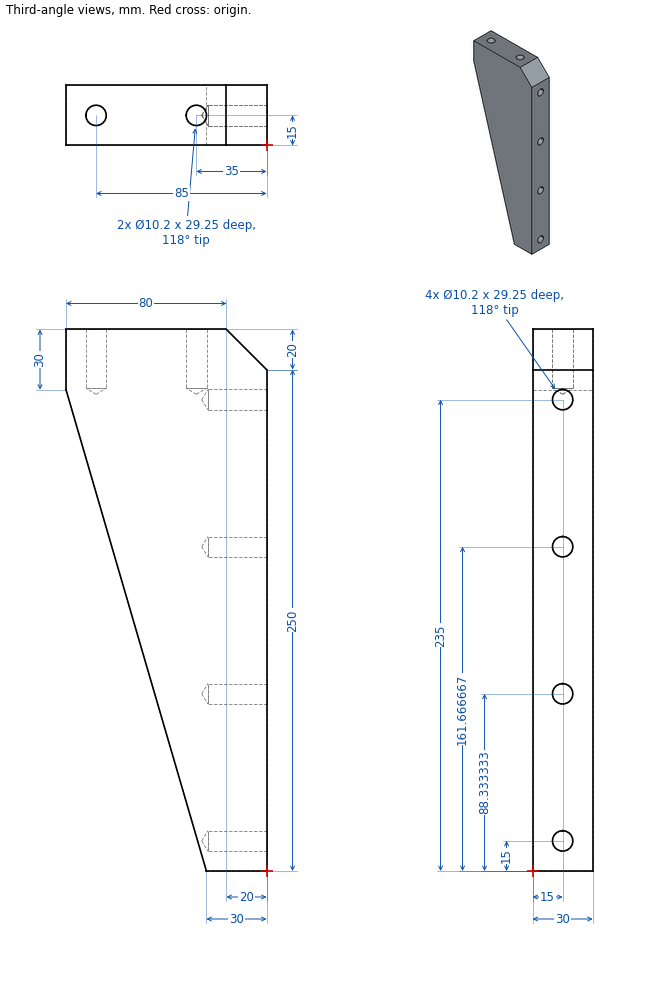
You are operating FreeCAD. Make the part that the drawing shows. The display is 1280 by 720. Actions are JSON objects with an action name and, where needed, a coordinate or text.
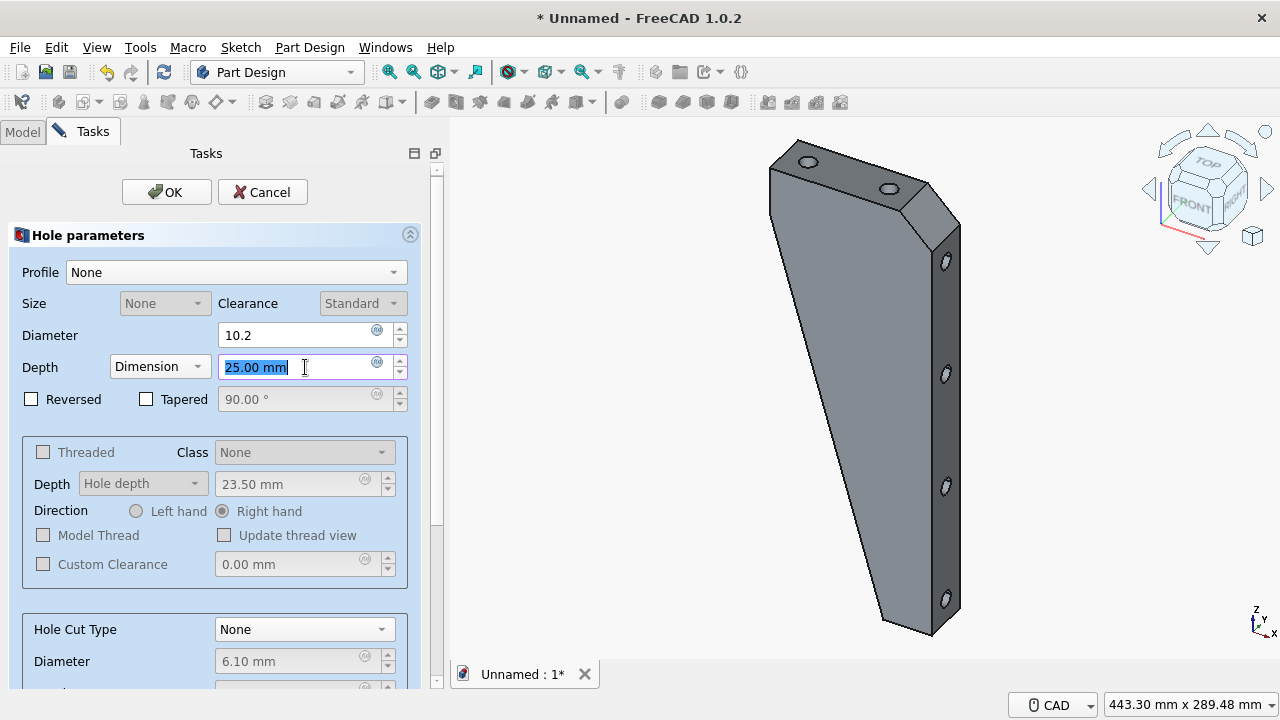
{"action": "type", "text": "29.25"}
{"action": "key", "text": "Tab"}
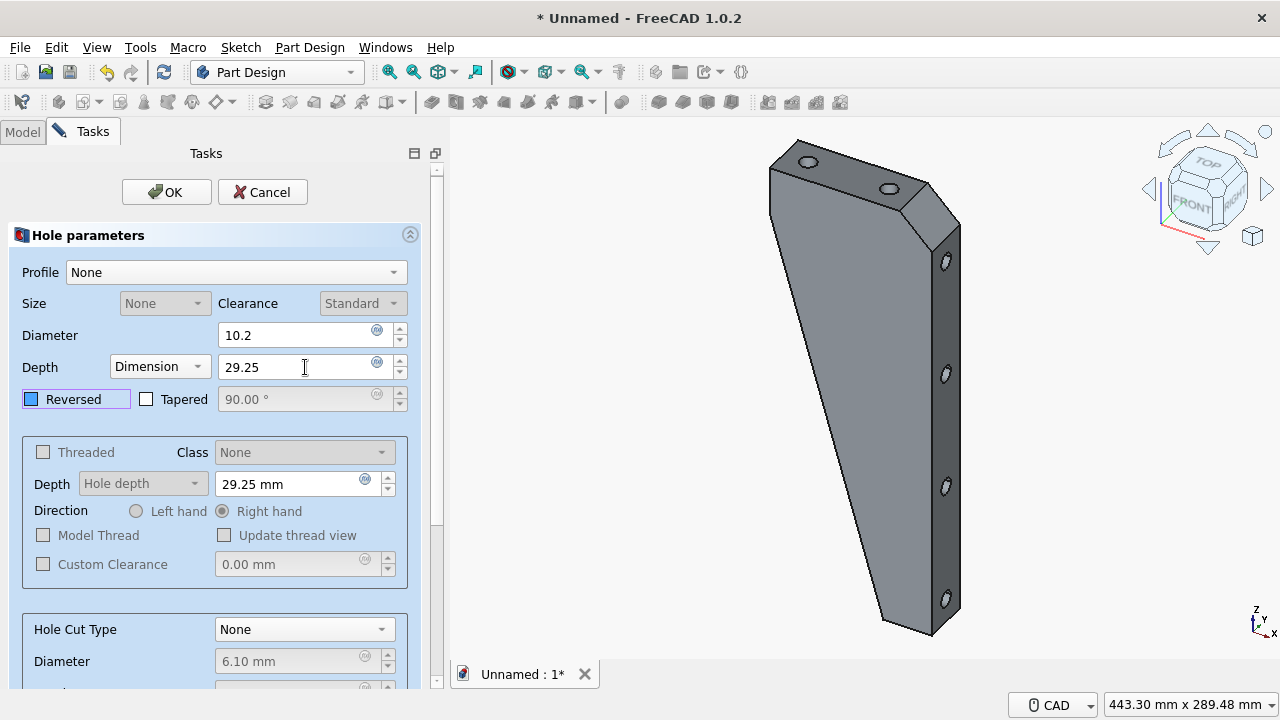
{"action": "left_click", "coordinate": [167, 192]}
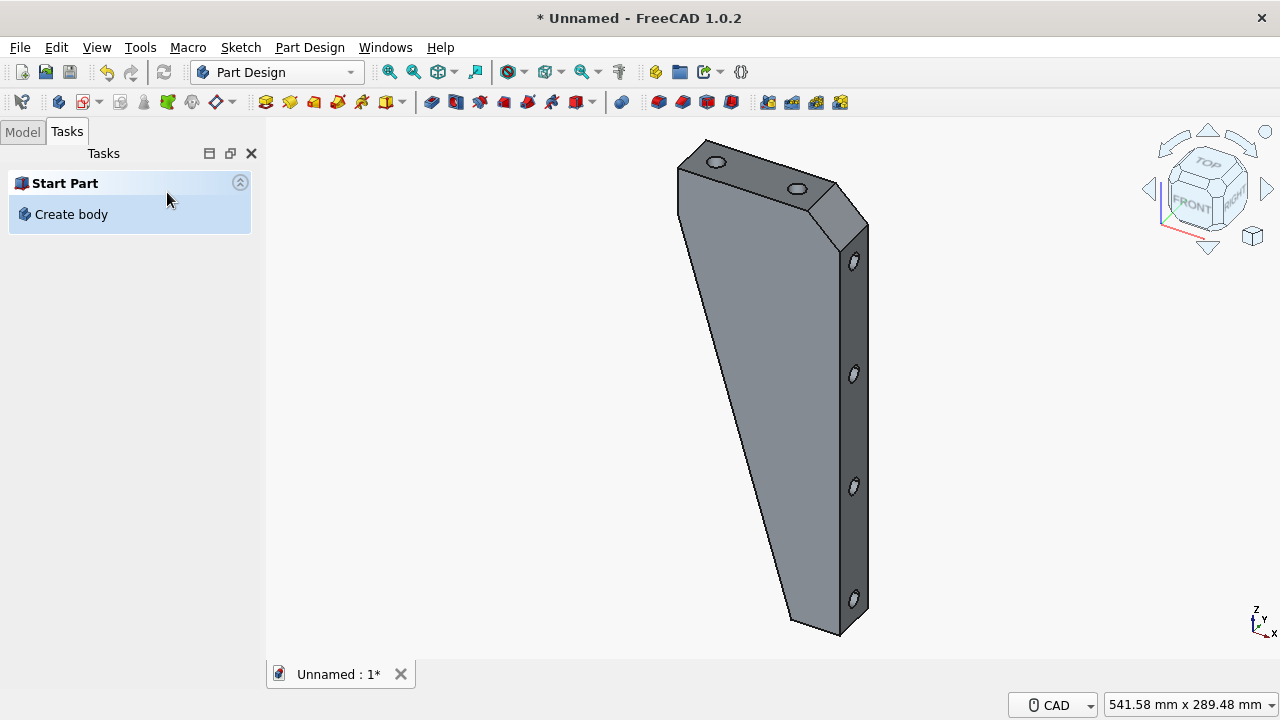
{"action": "key", "text": "0"}